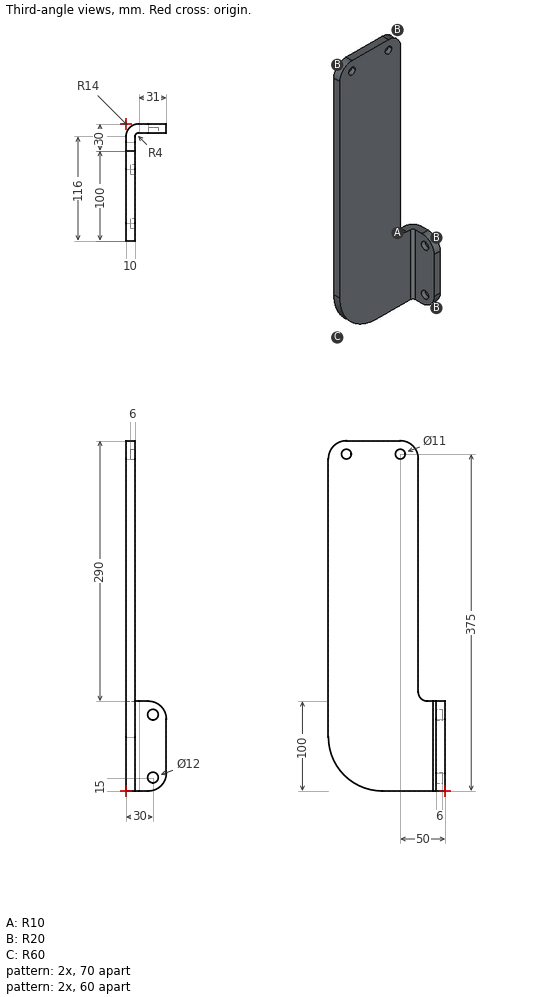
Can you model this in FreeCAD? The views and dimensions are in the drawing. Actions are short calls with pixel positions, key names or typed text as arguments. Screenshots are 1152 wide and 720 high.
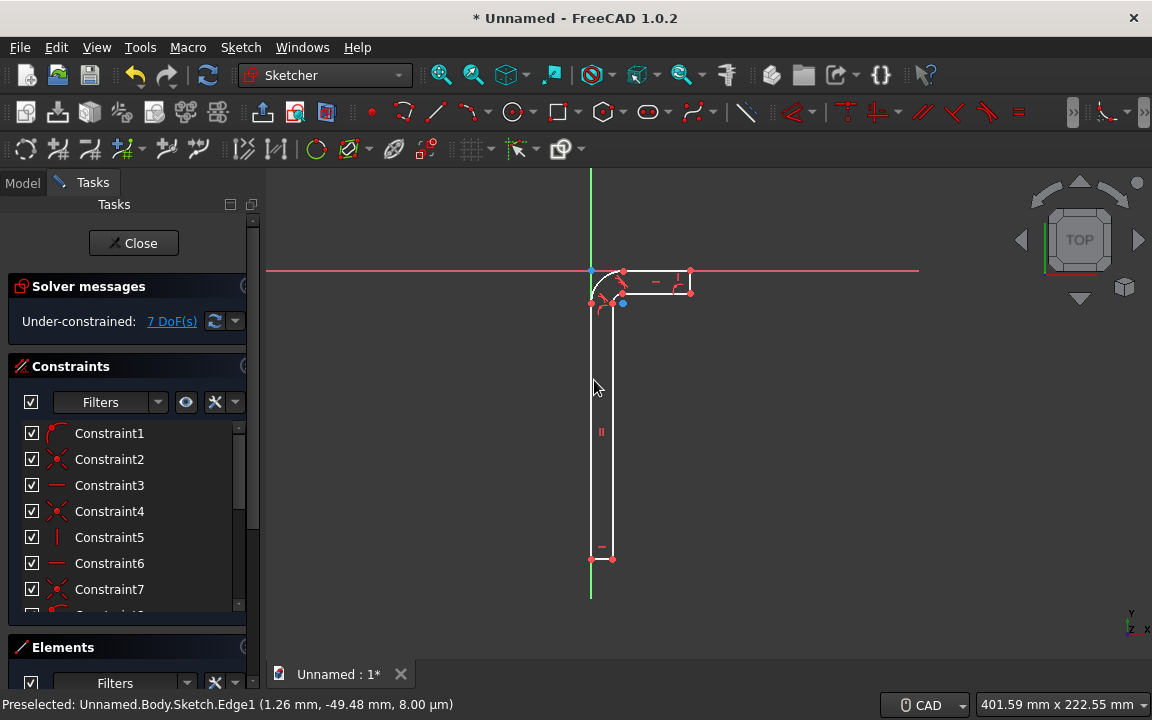
click(670, 271)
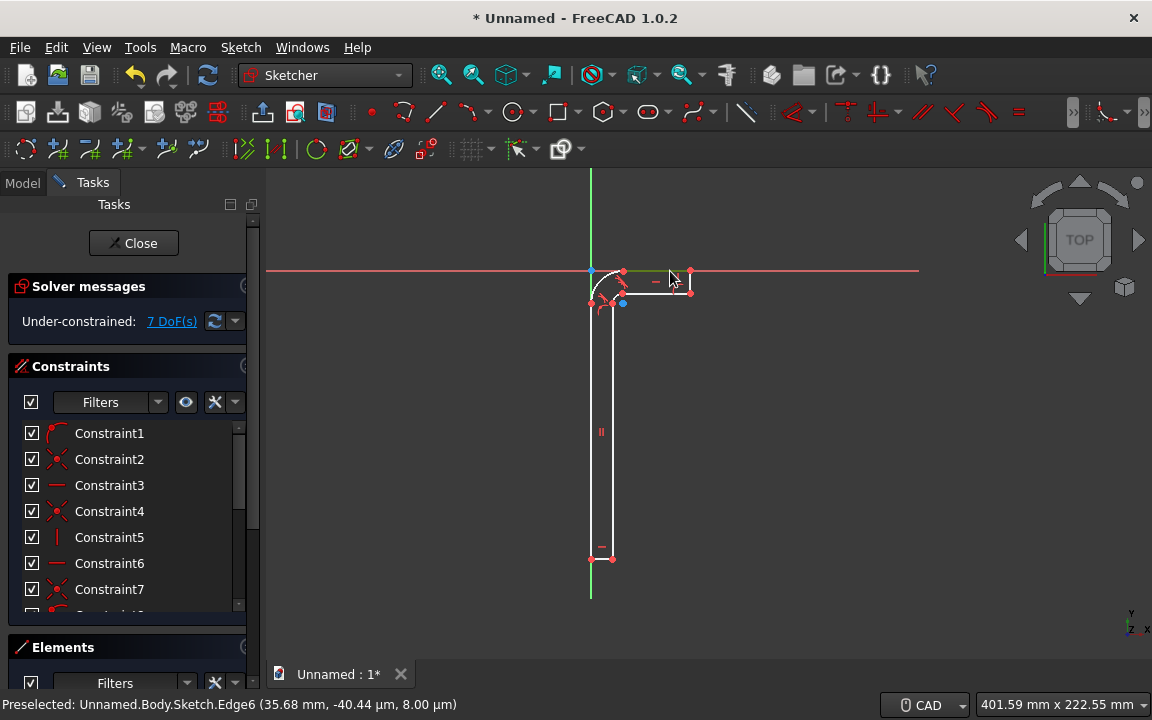
key(h)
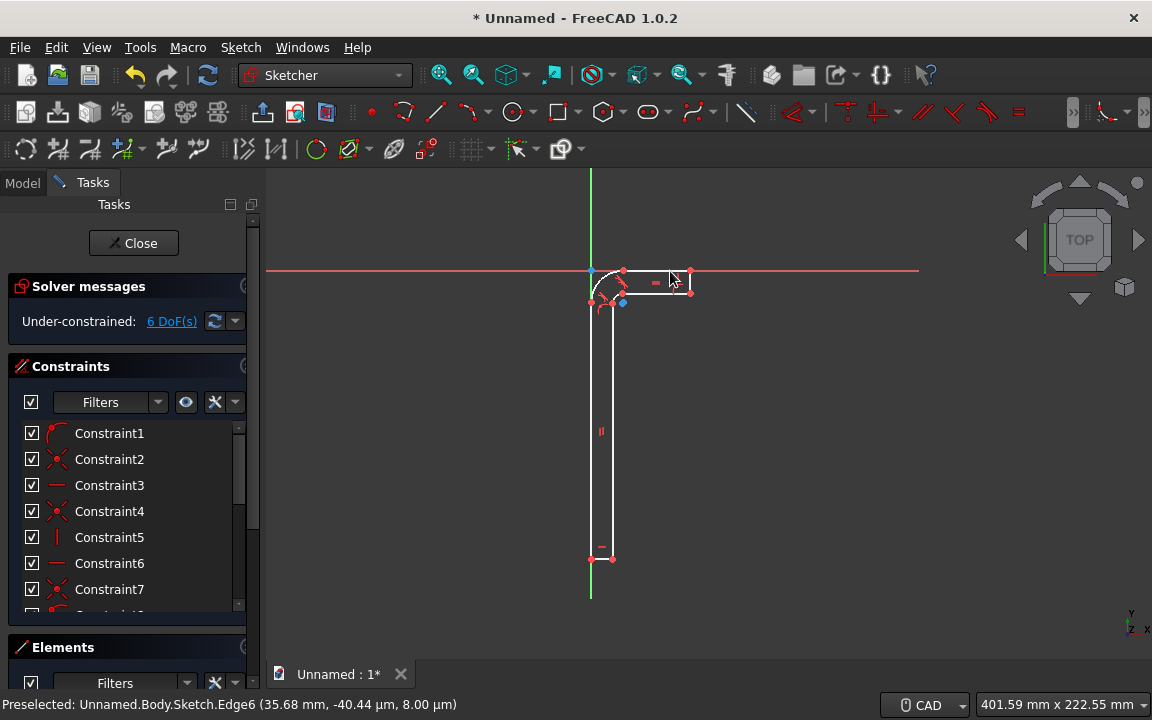
scroll(616, 297, up, 4)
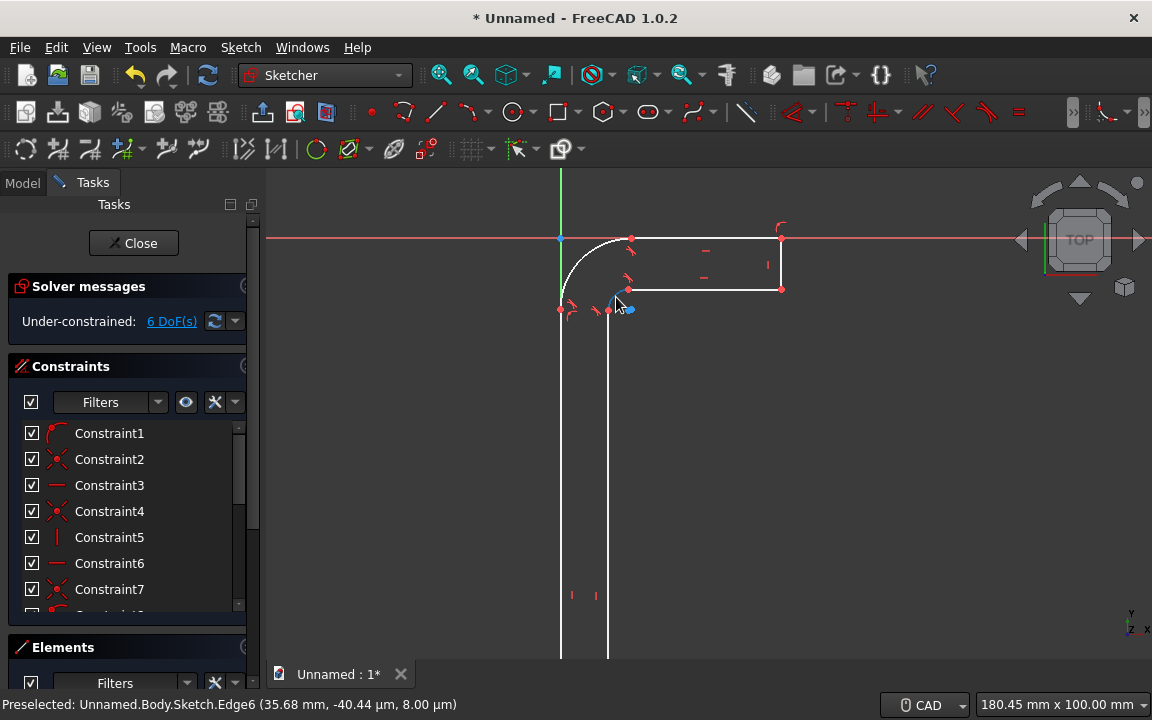
click(614, 296)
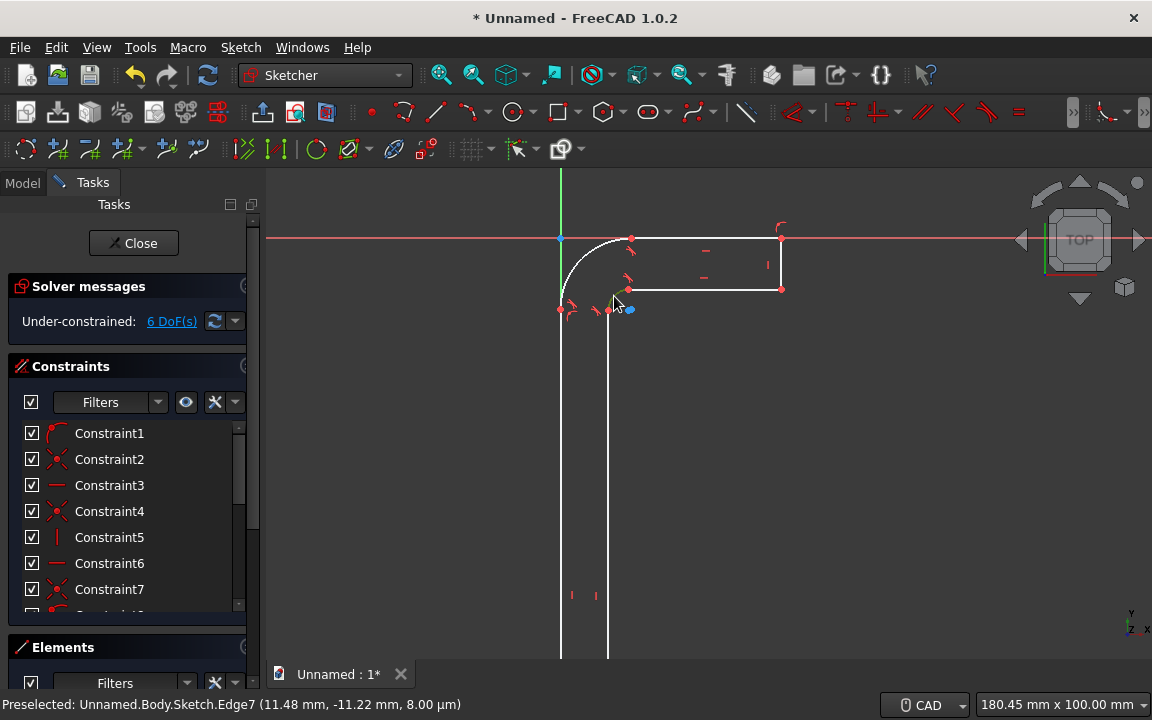
click(581, 259)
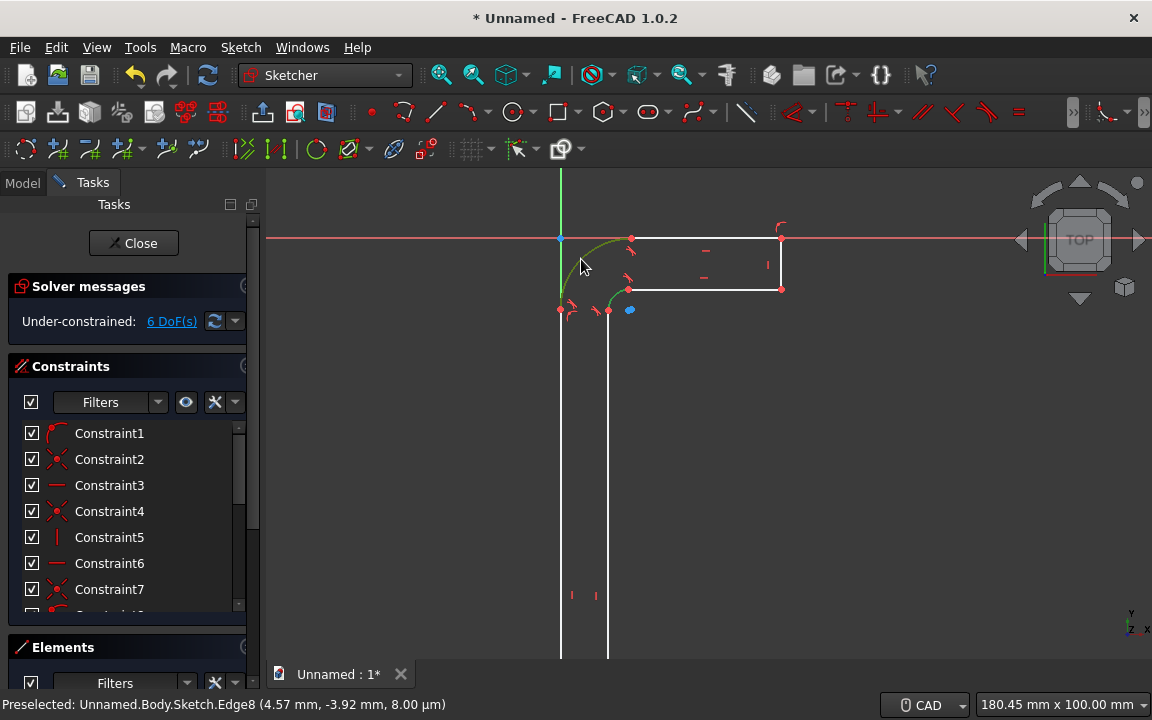
click(846, 112)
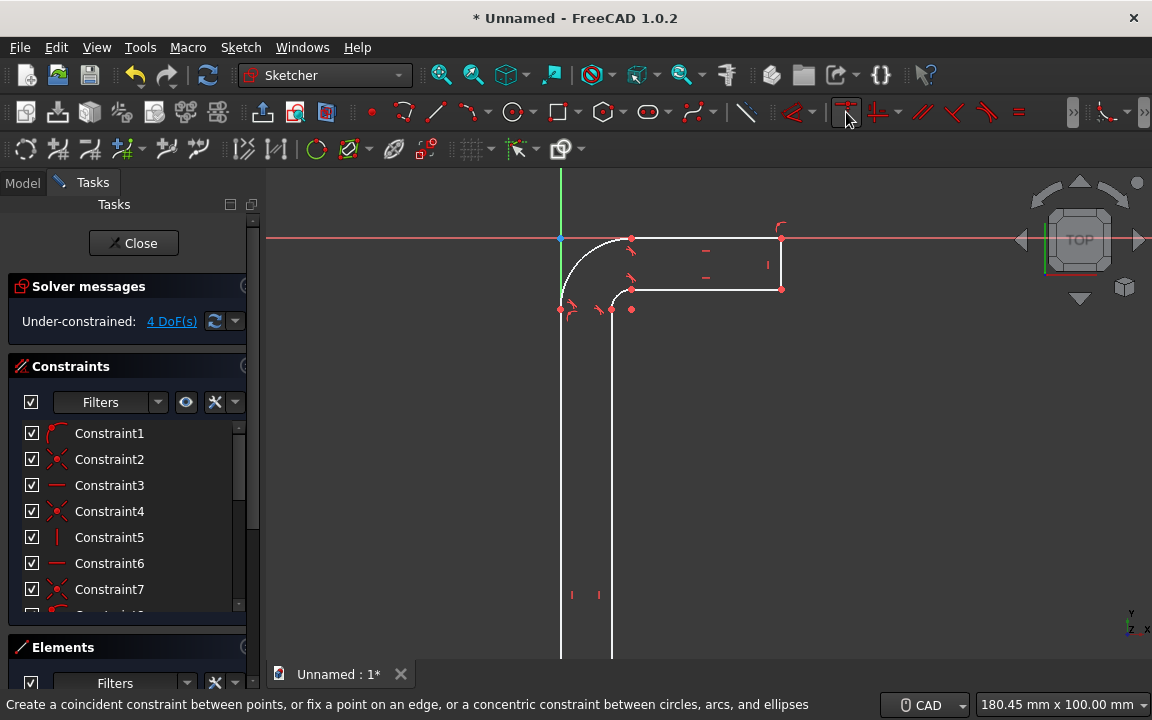
click(792, 112)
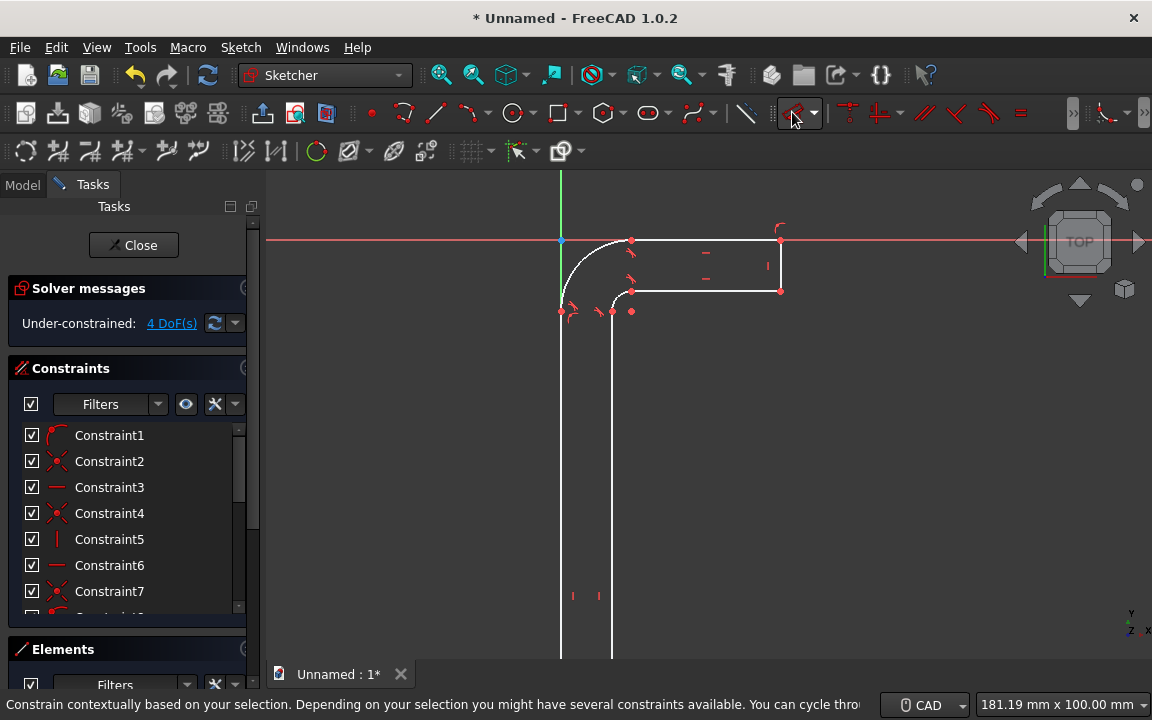
scroll(623, 293, up, 4)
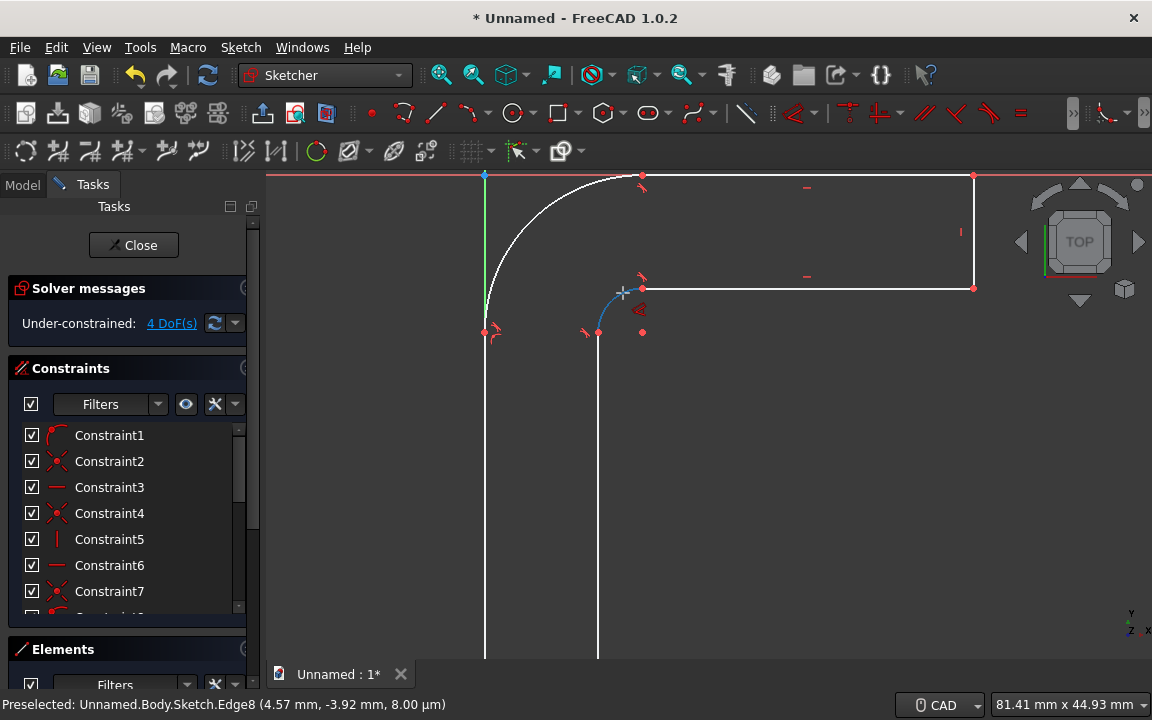
click(622, 293)
click(607, 265)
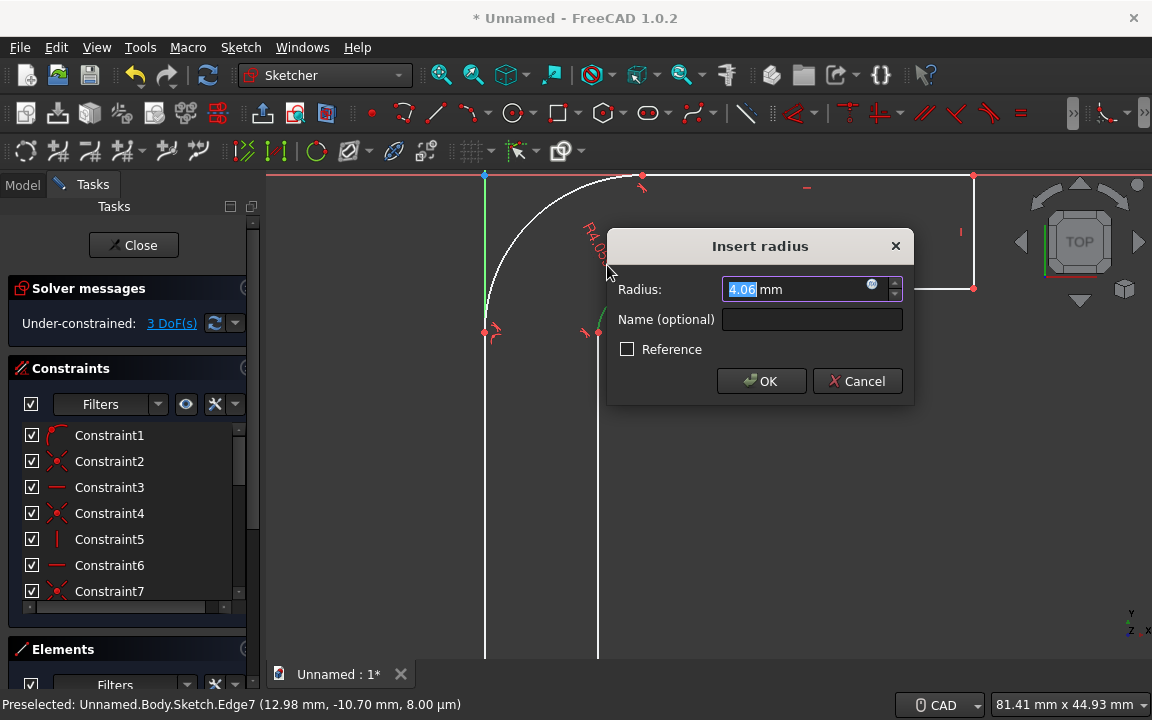
text(4)
key(Return)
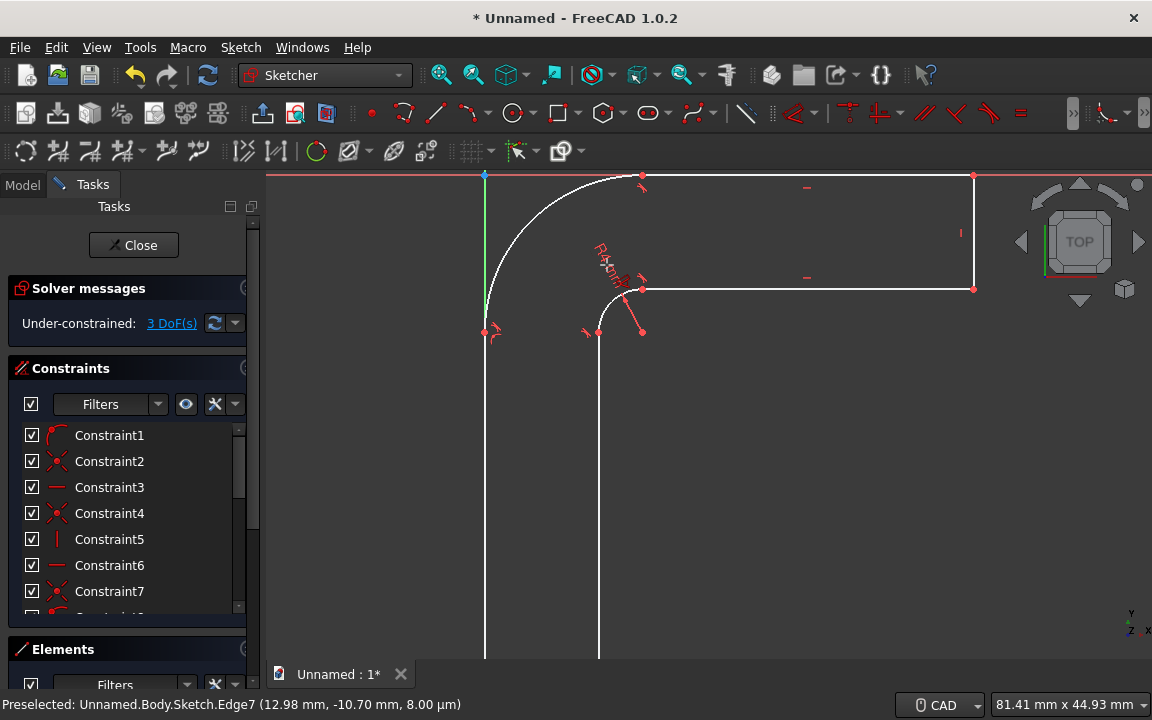
click(502, 261)
click(453, 338)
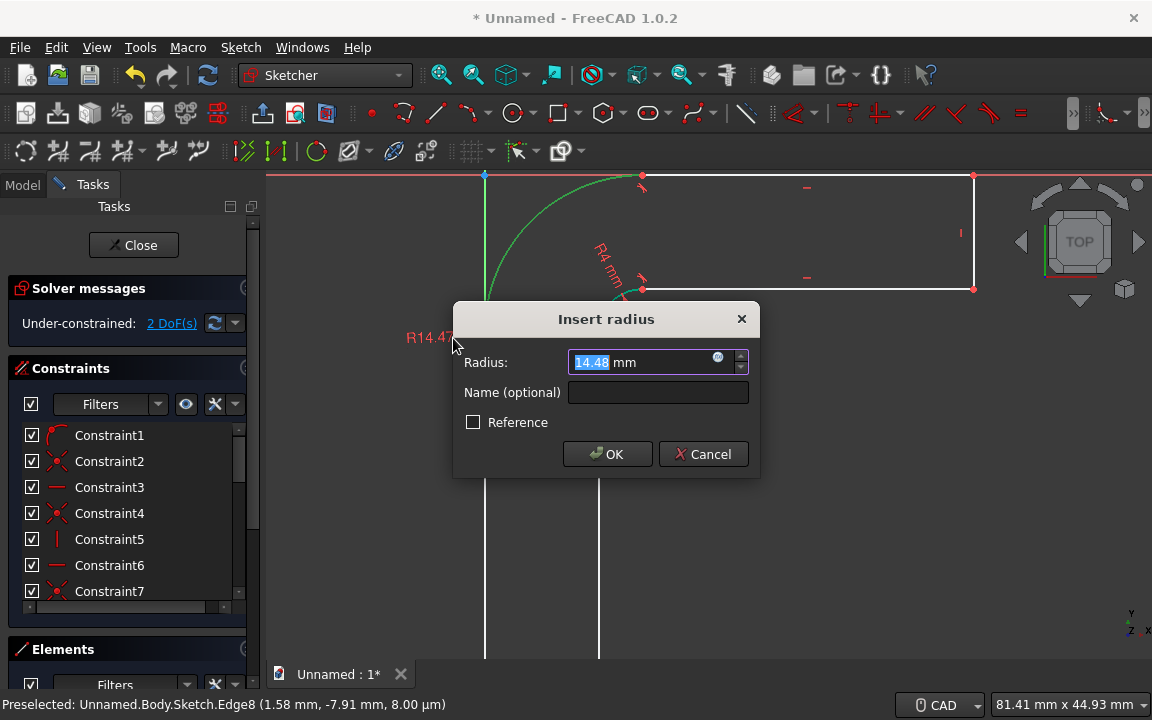
text(14)
key(Return)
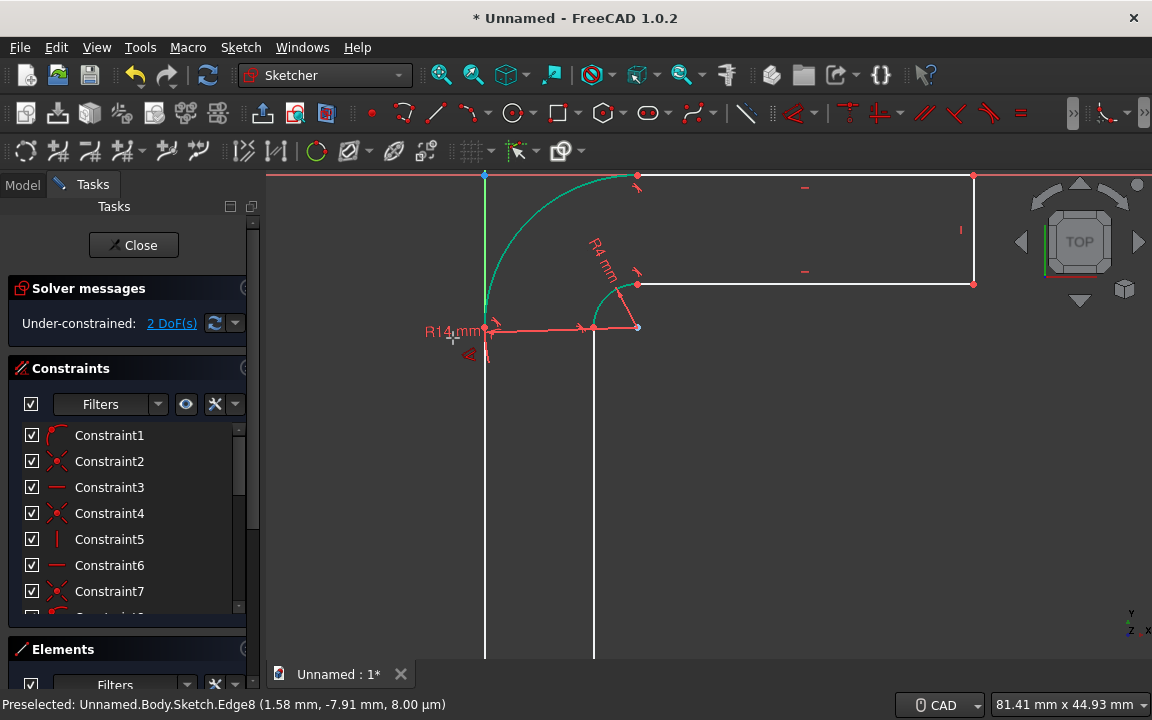
scroll(618, 296, down, 8)